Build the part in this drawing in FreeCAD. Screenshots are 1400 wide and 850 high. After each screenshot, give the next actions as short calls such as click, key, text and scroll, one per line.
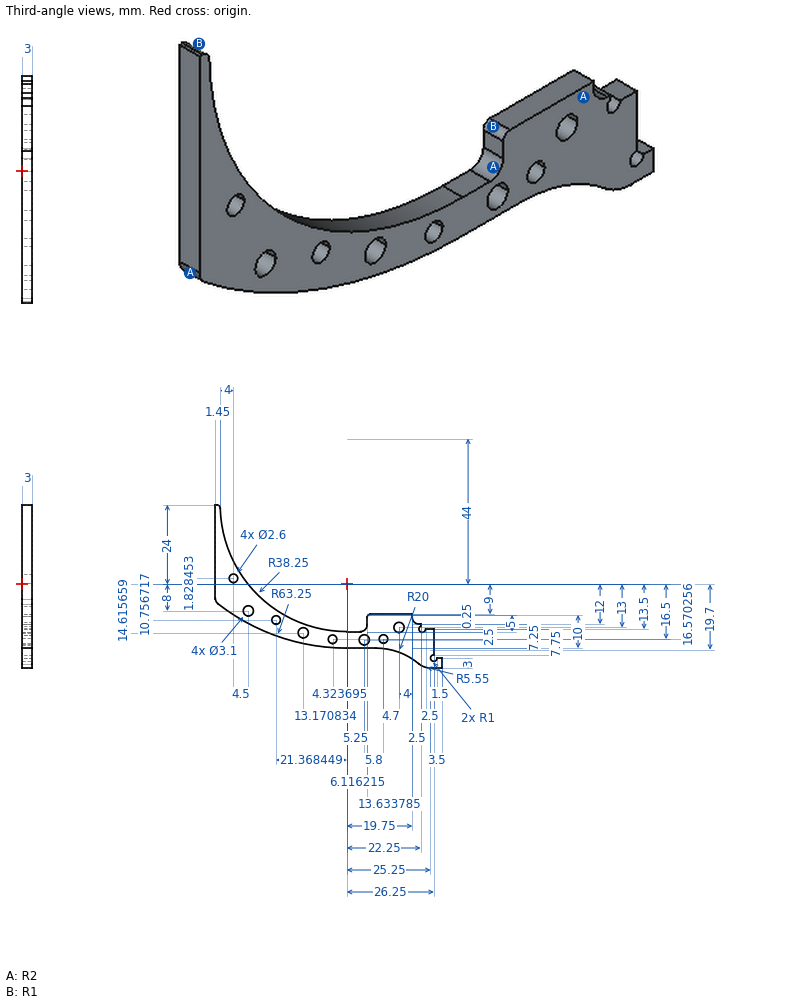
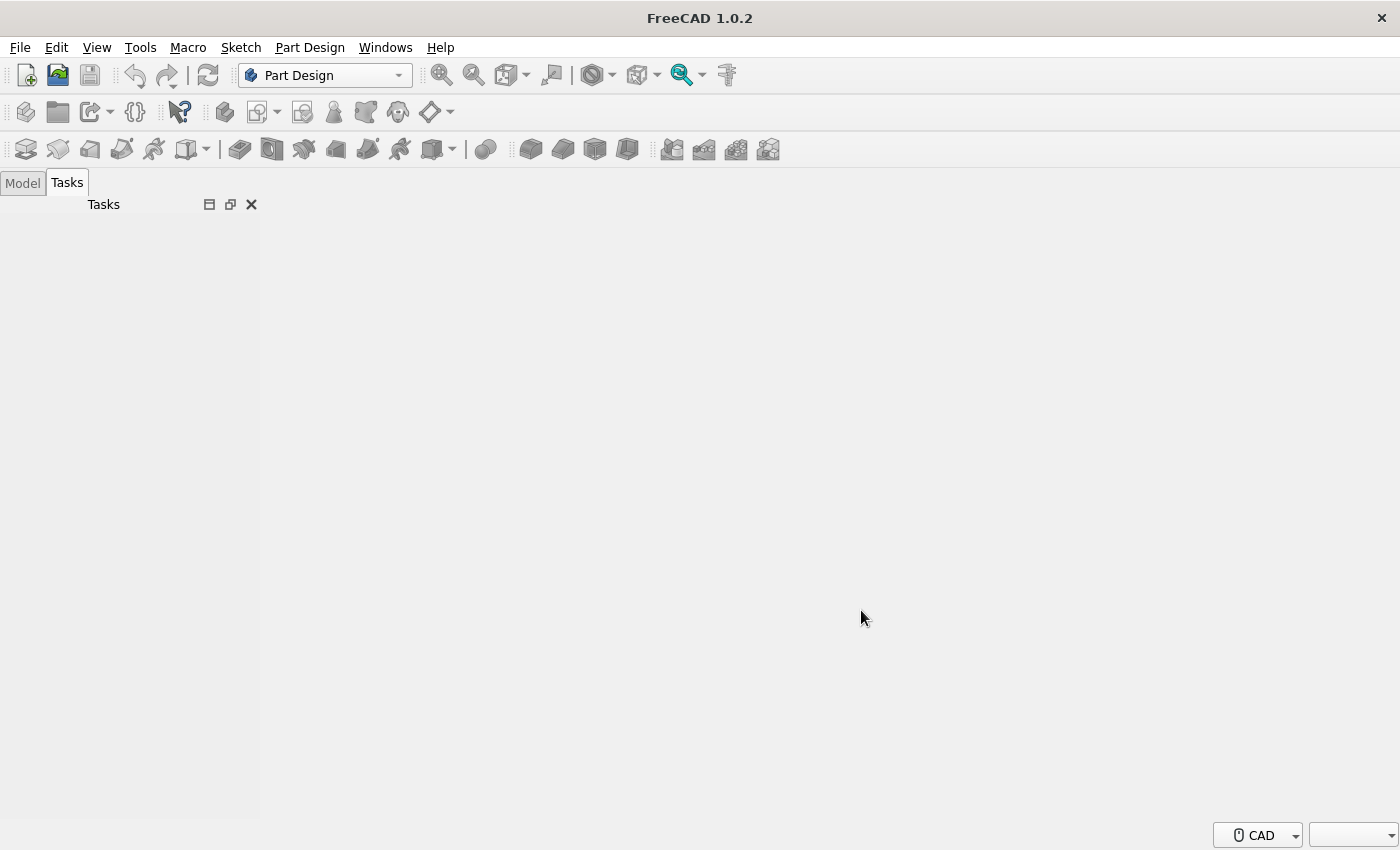
key(ctrl+n)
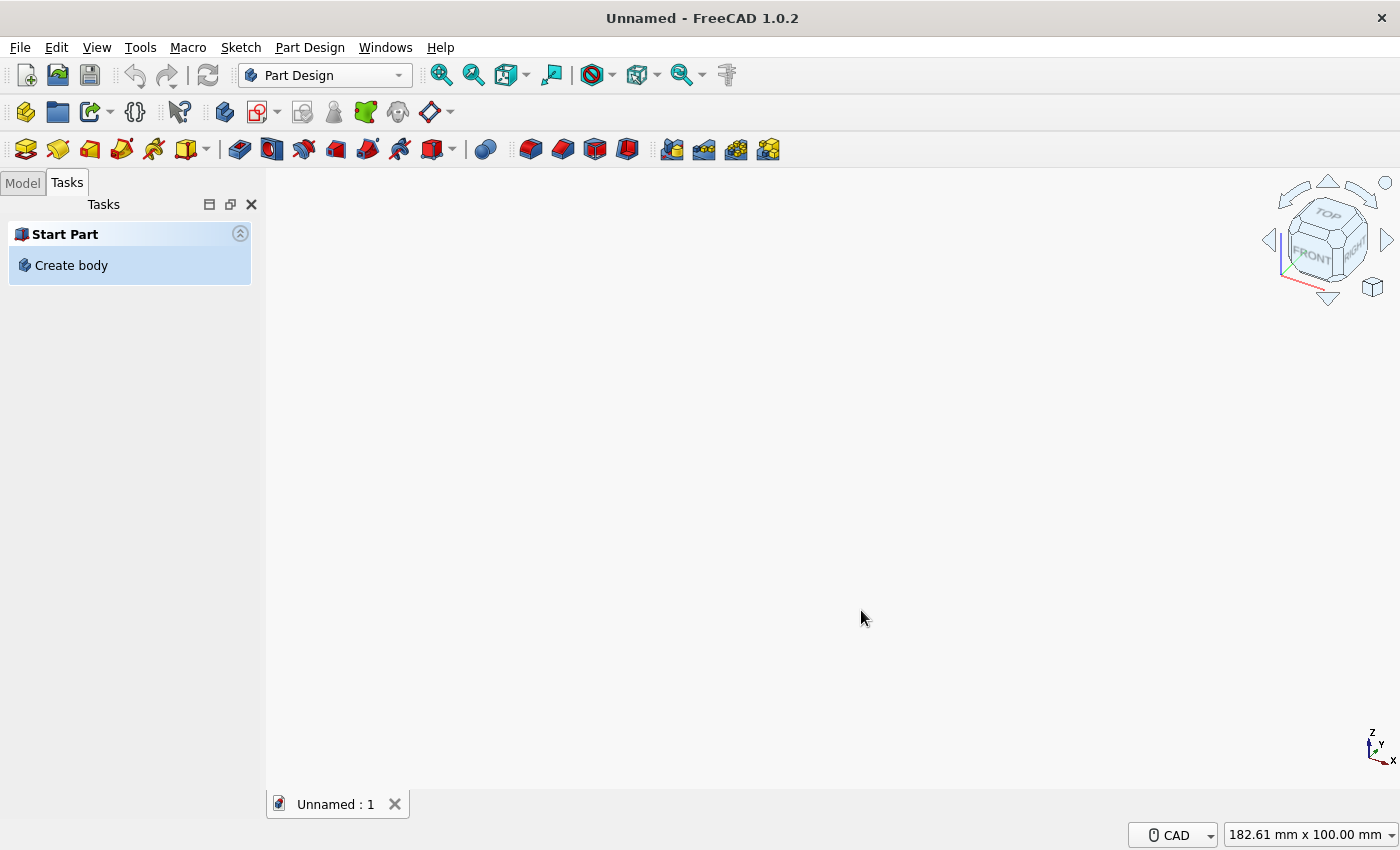
click(258, 112)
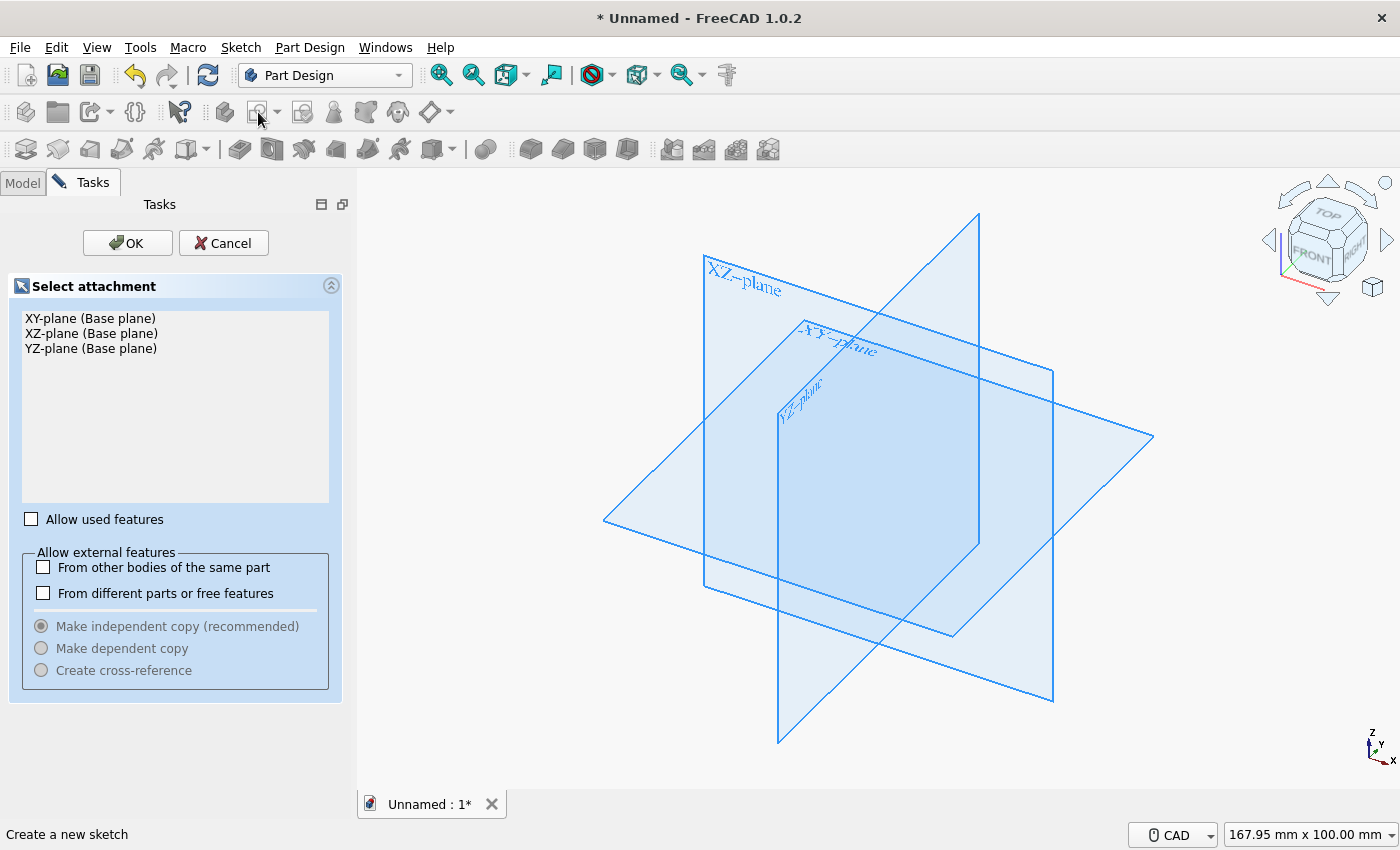
click(82, 348)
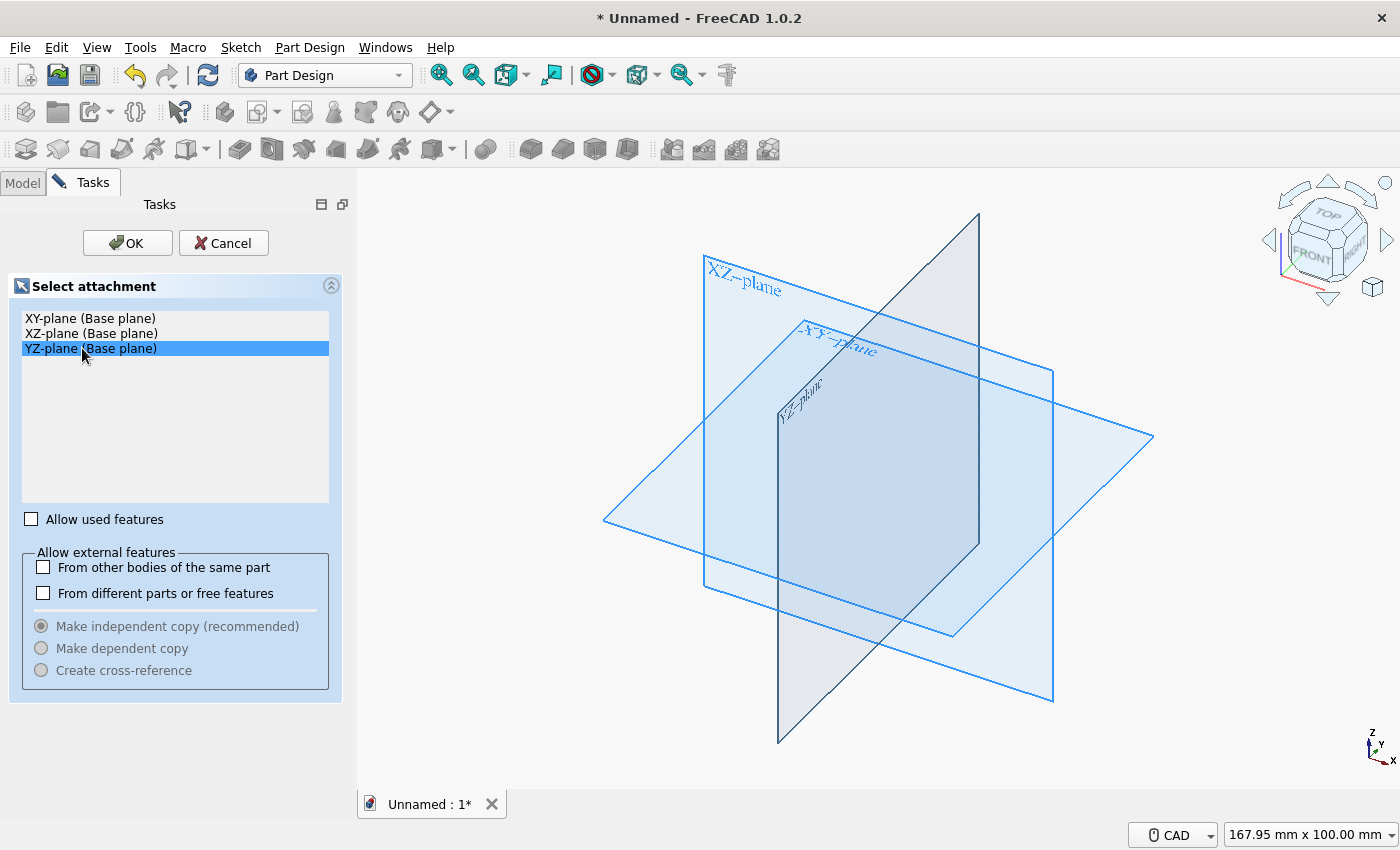
click(128, 243)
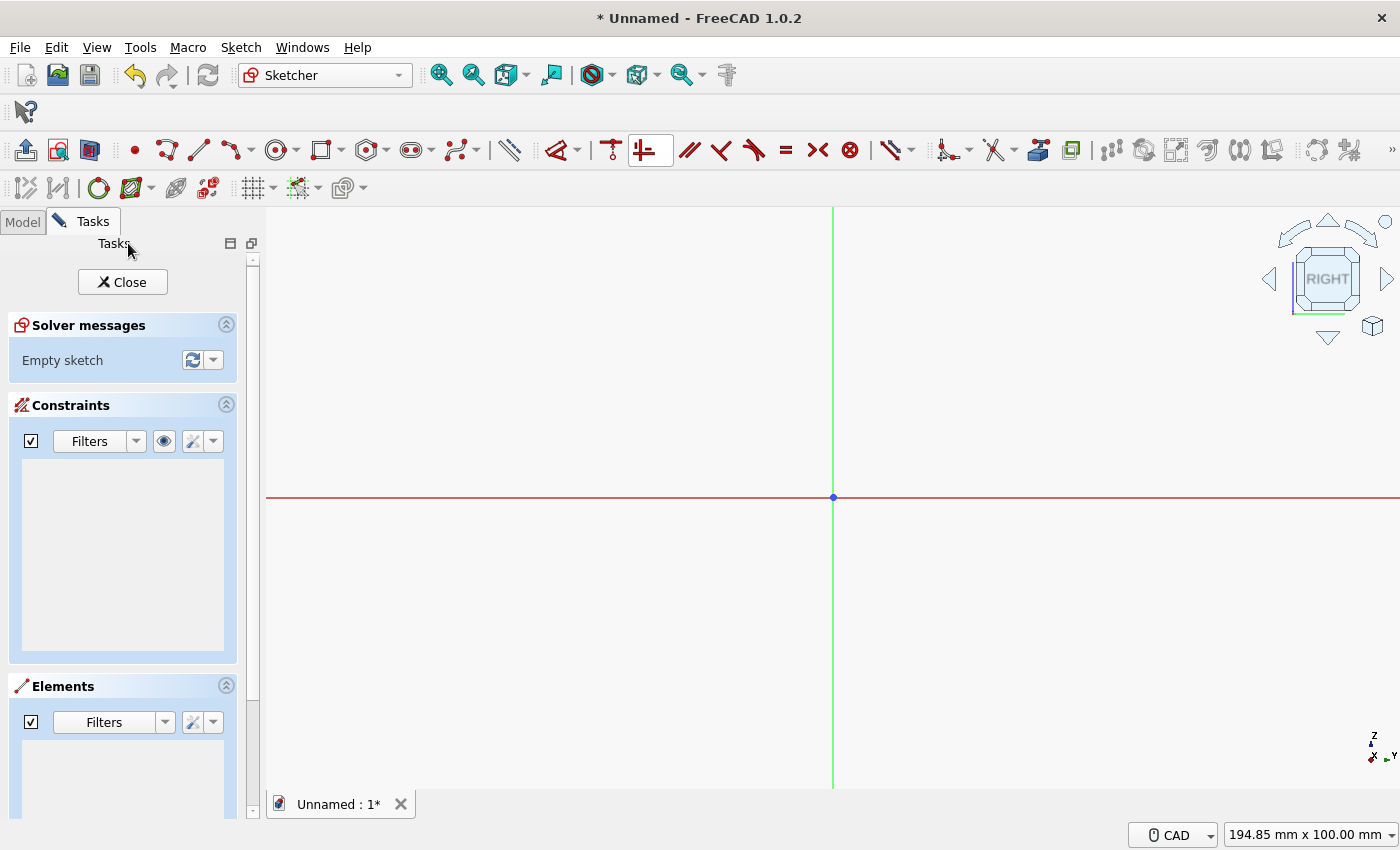
scroll(796, 456, up, 2)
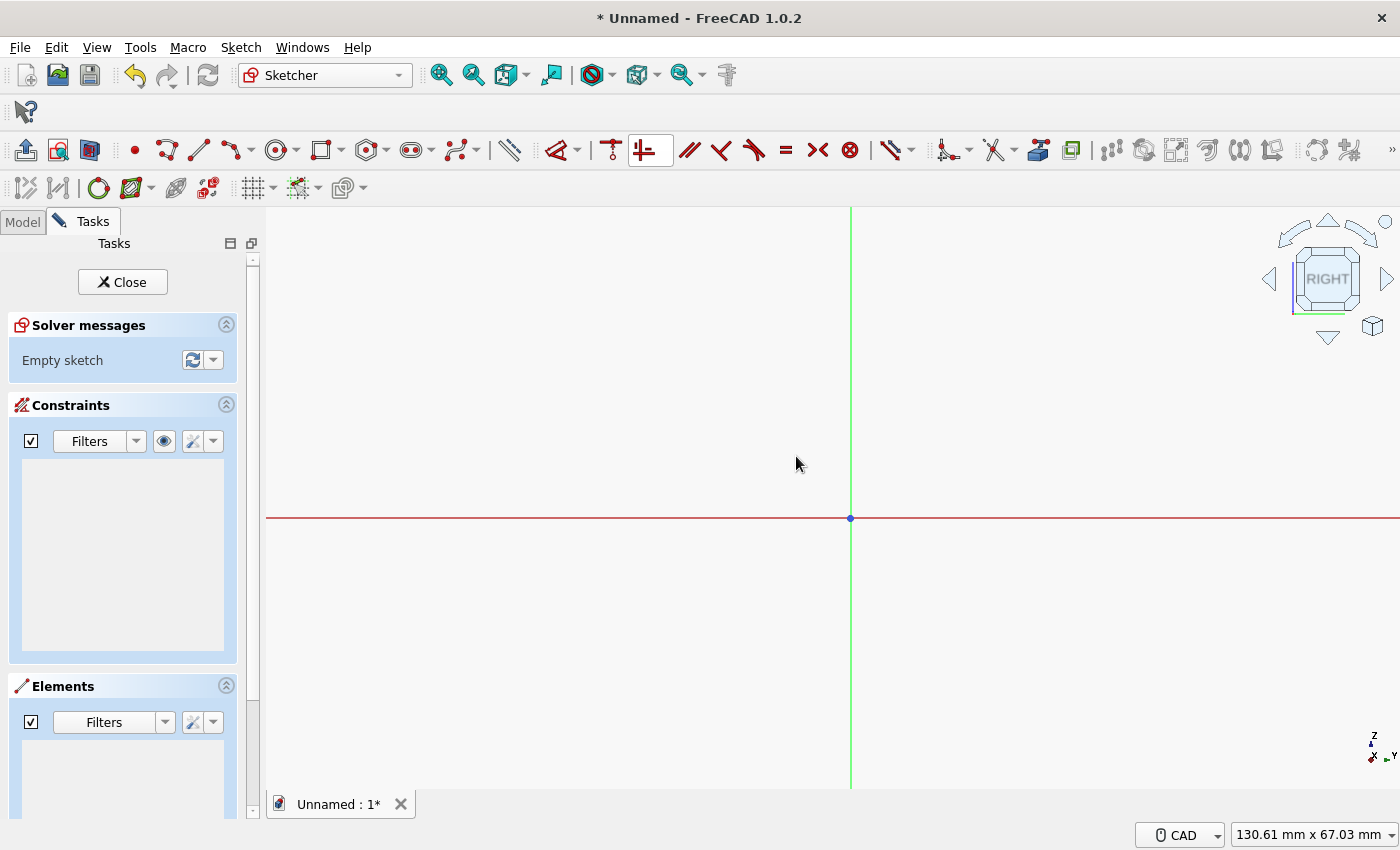
key(g)
key(m)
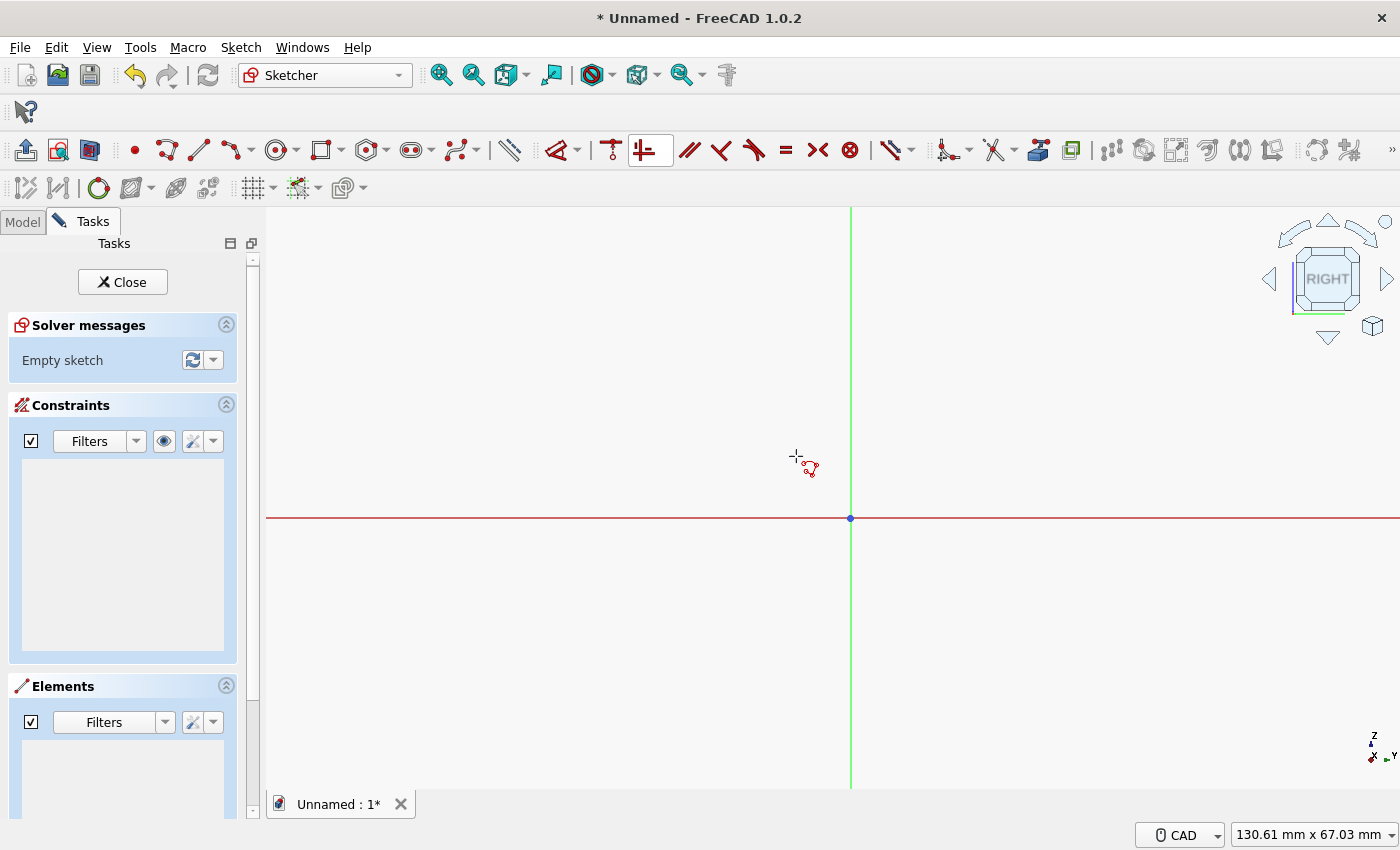
click(519, 310)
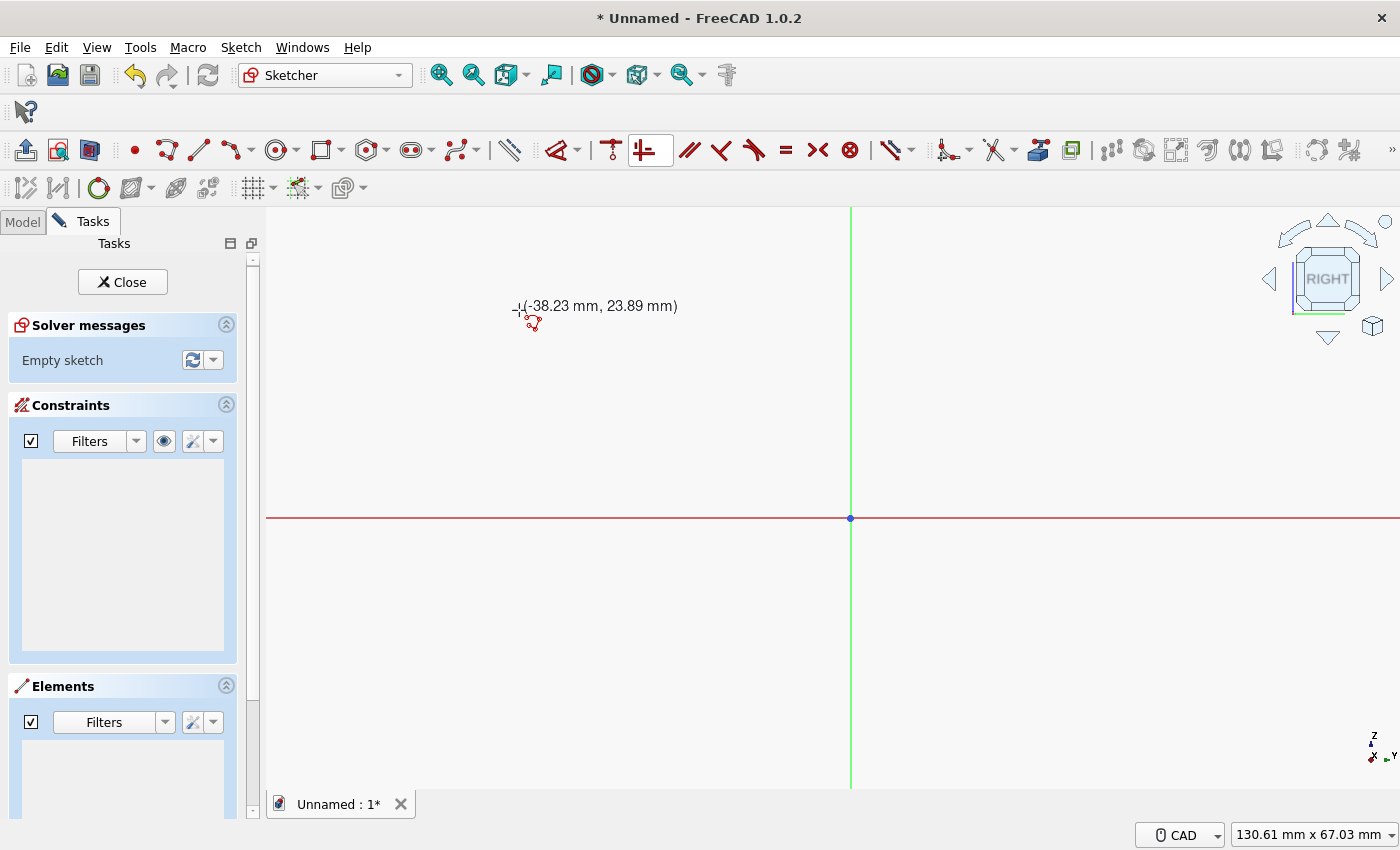
scroll(506, 310, up, 2)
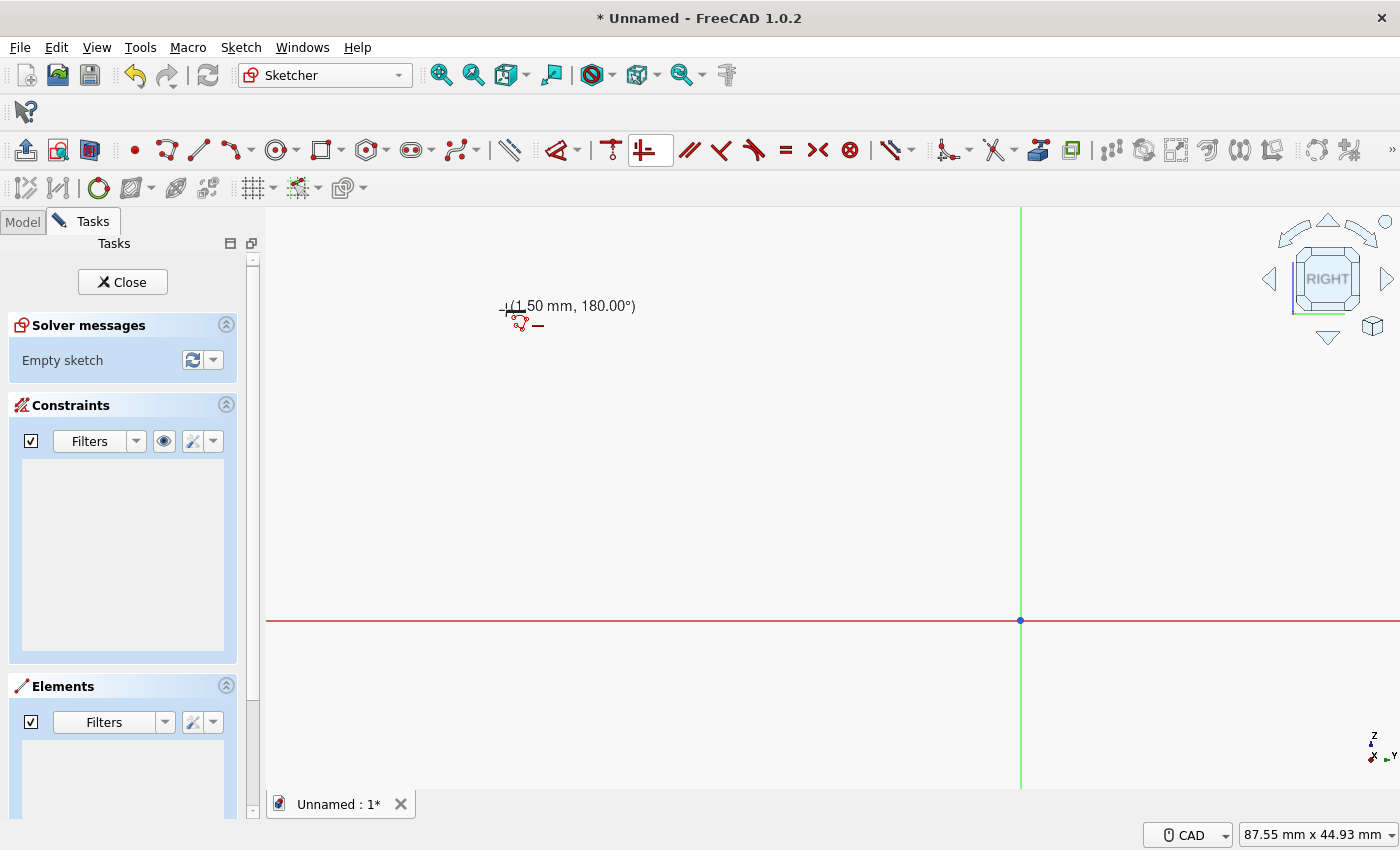
click(506, 310)
click(506, 689)
right_click(506, 689)